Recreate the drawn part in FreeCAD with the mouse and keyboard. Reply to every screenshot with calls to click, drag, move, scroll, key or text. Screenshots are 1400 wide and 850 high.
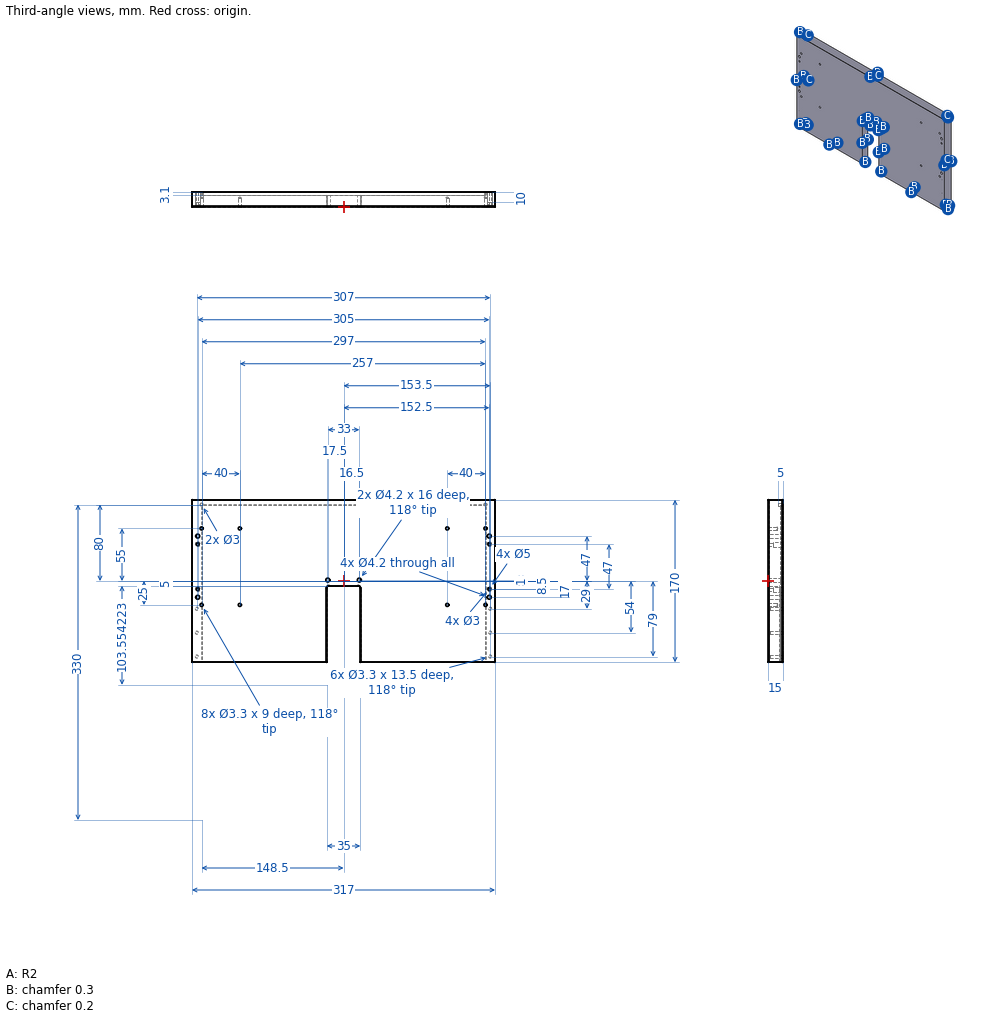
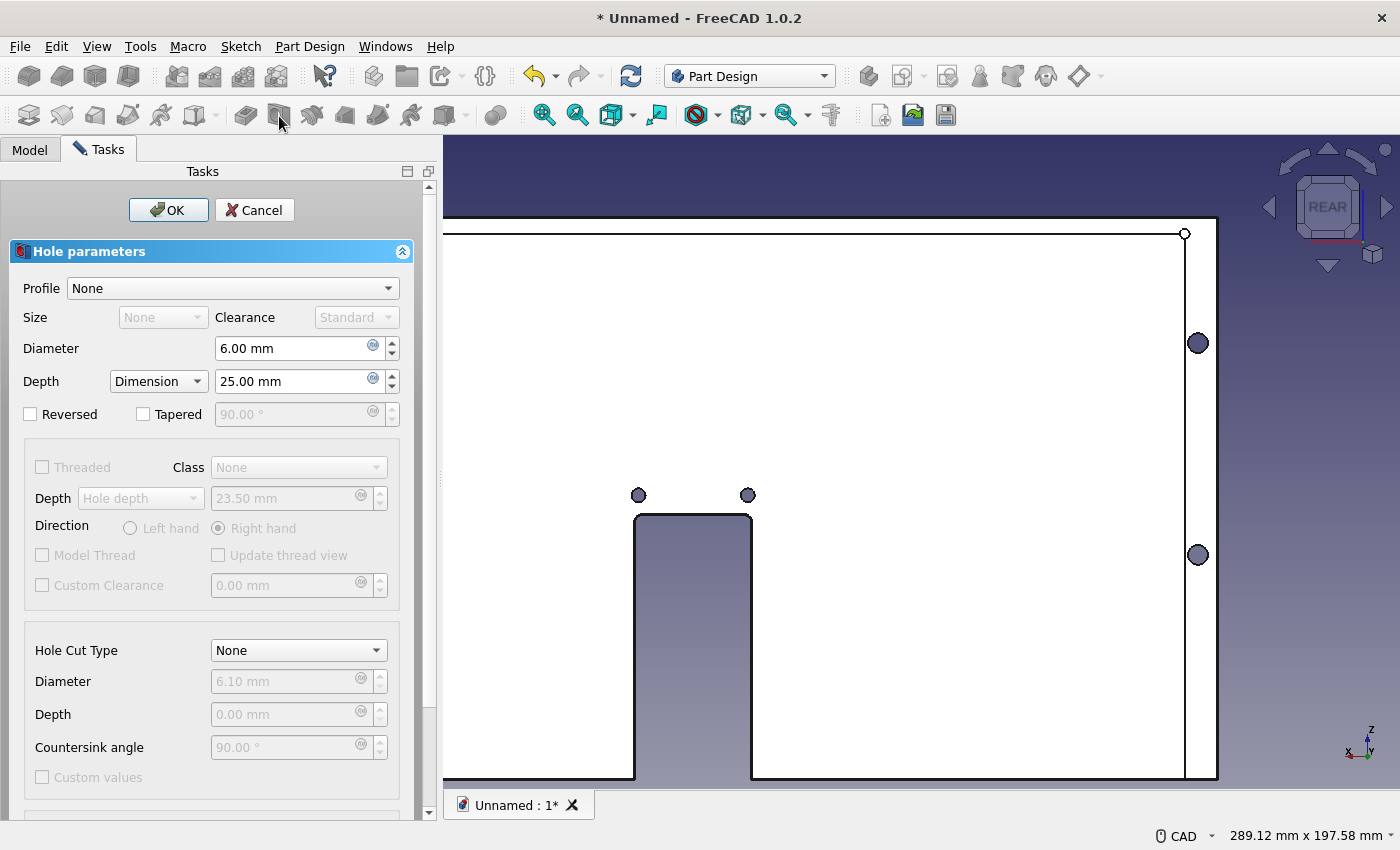
triple_click(300, 348)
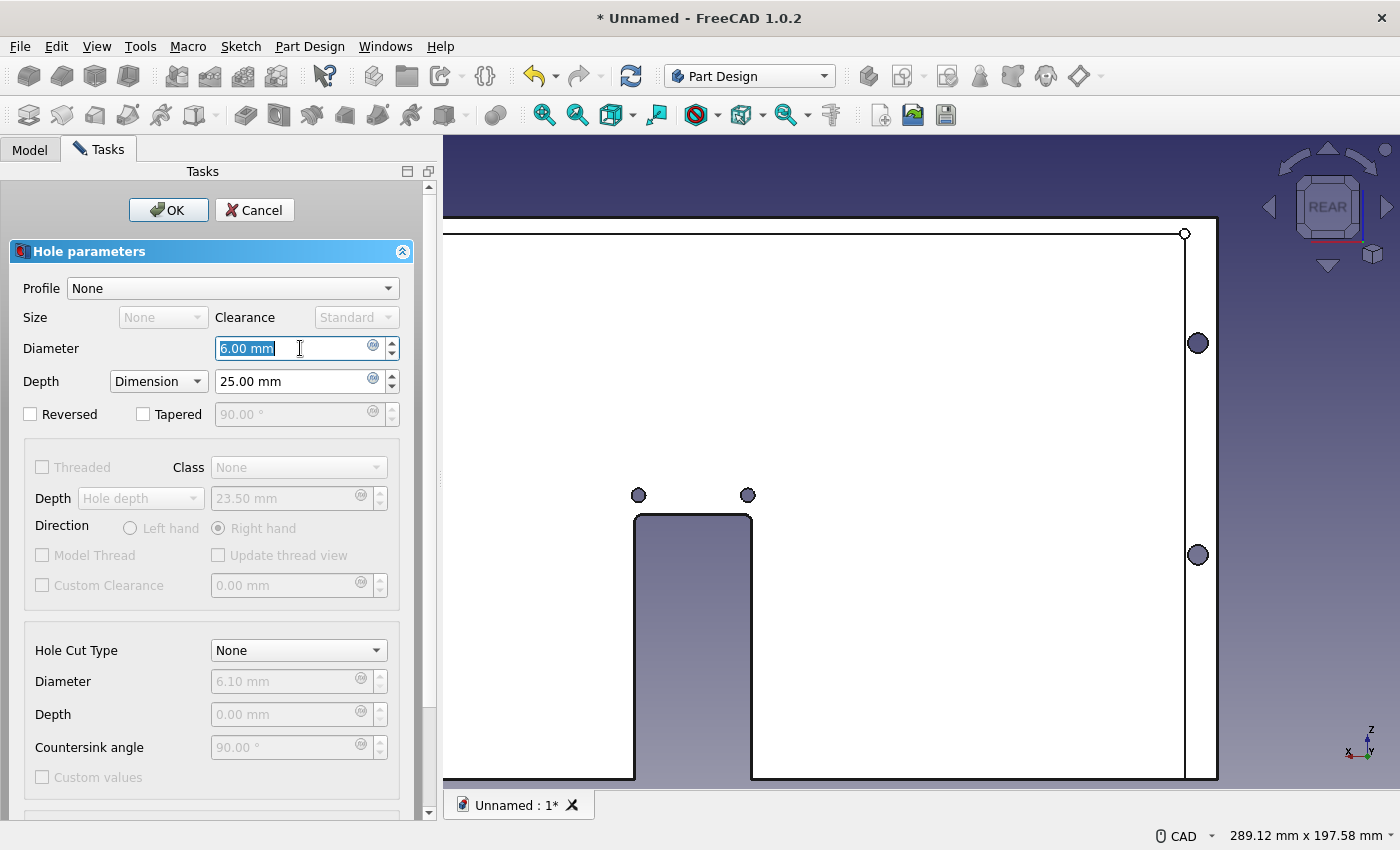
text(4.2)
key(Tab)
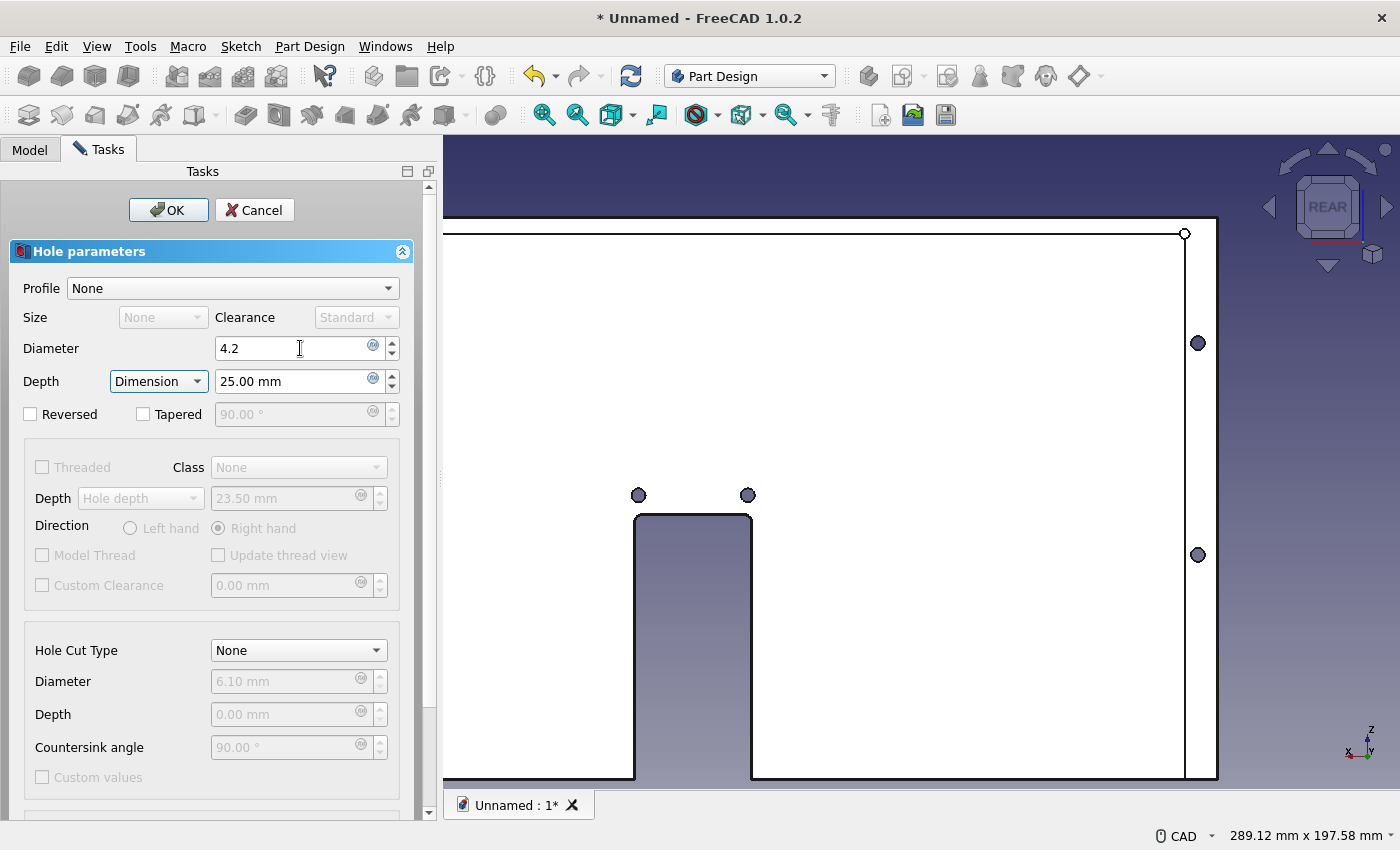
click(160, 382)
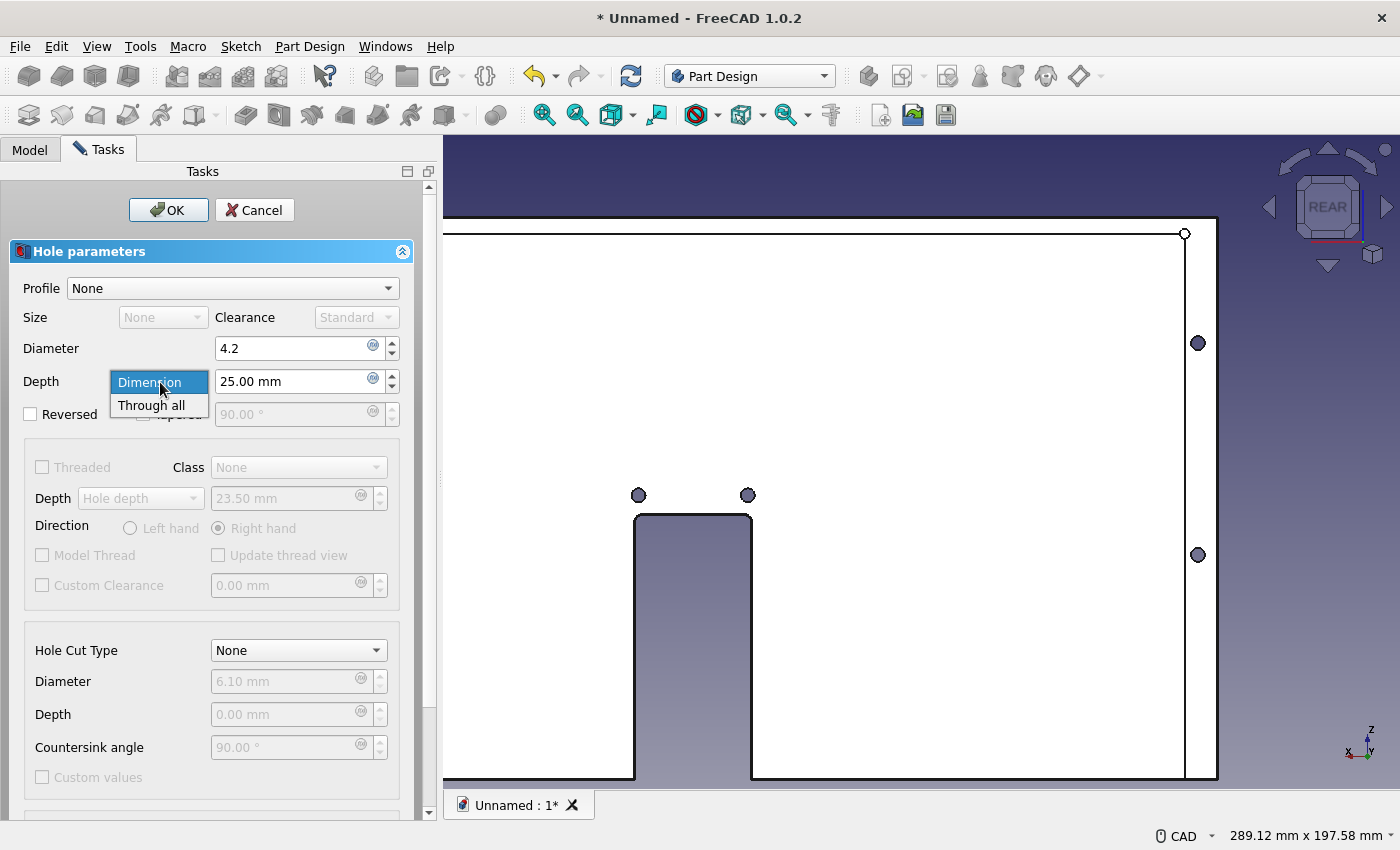
click(158, 406)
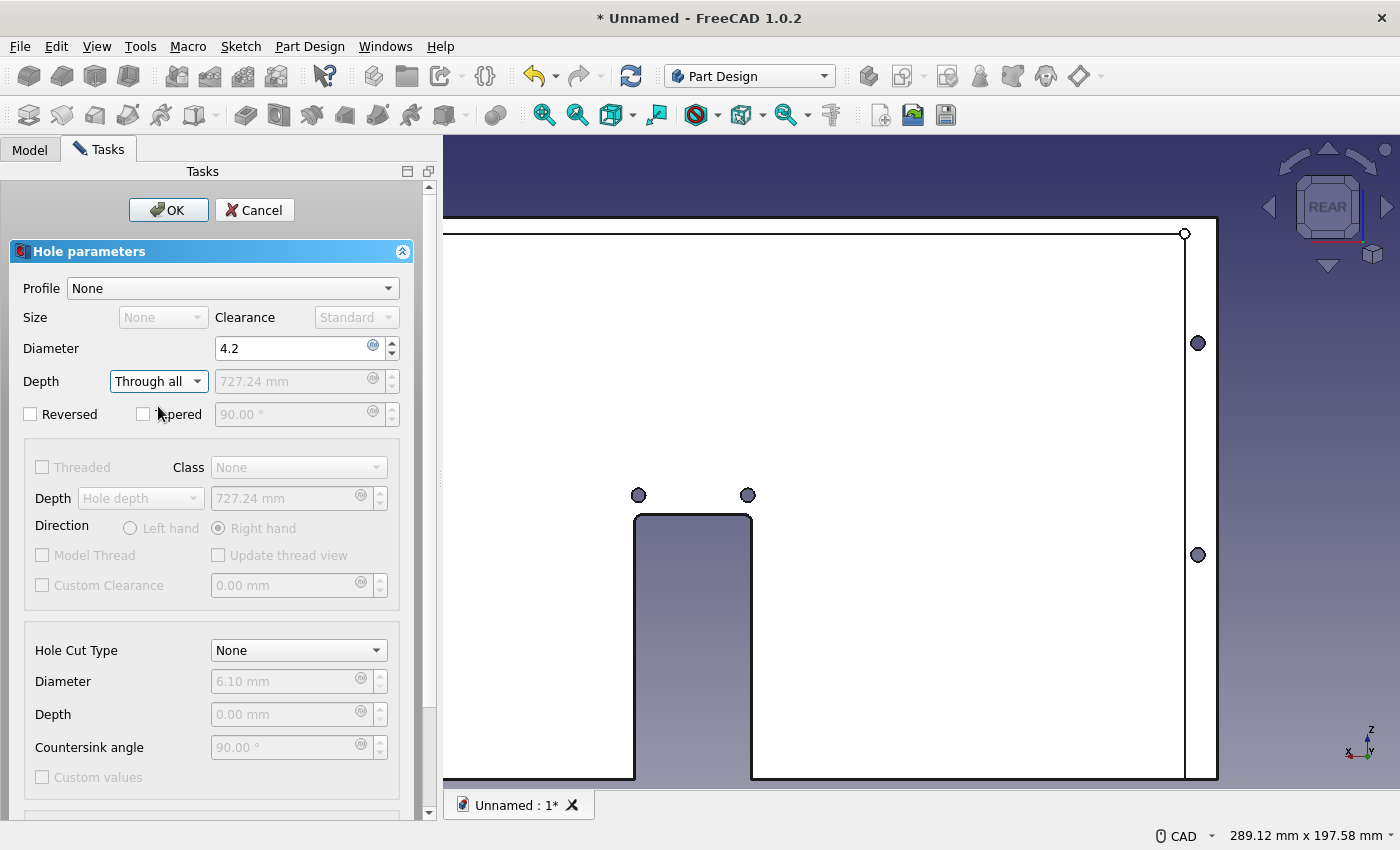
click(169, 210)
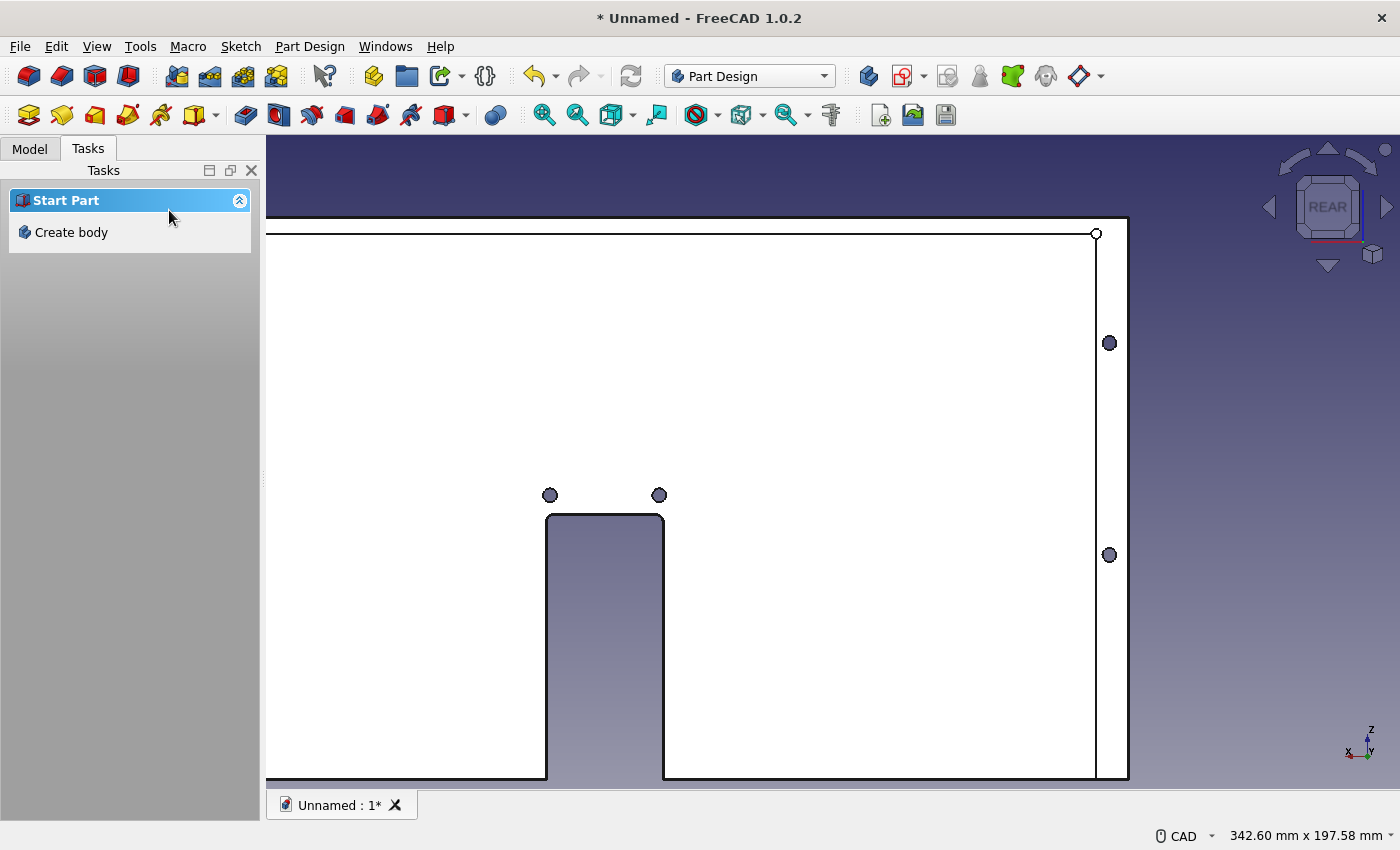
key(v)
key(f)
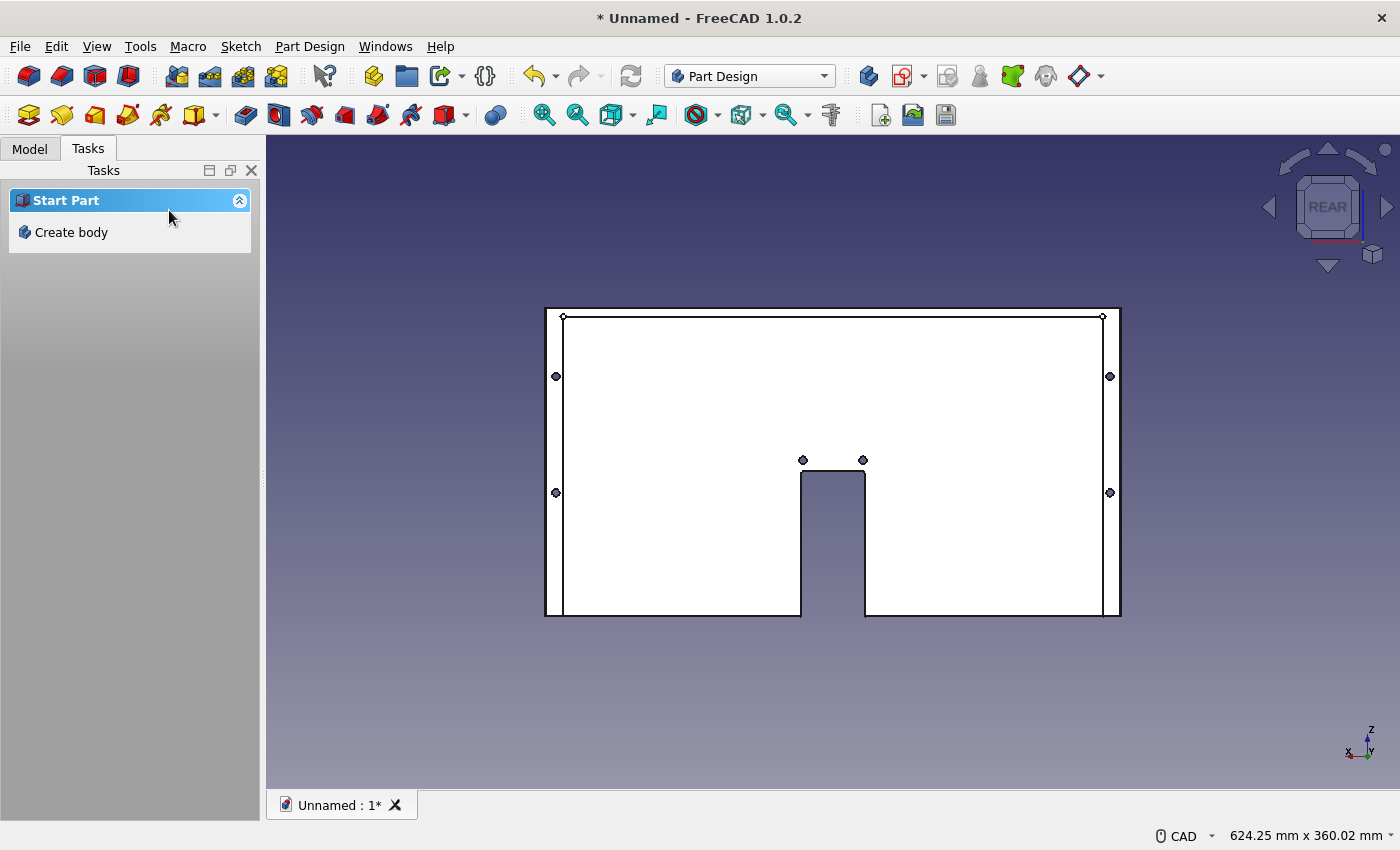
click(1111, 452)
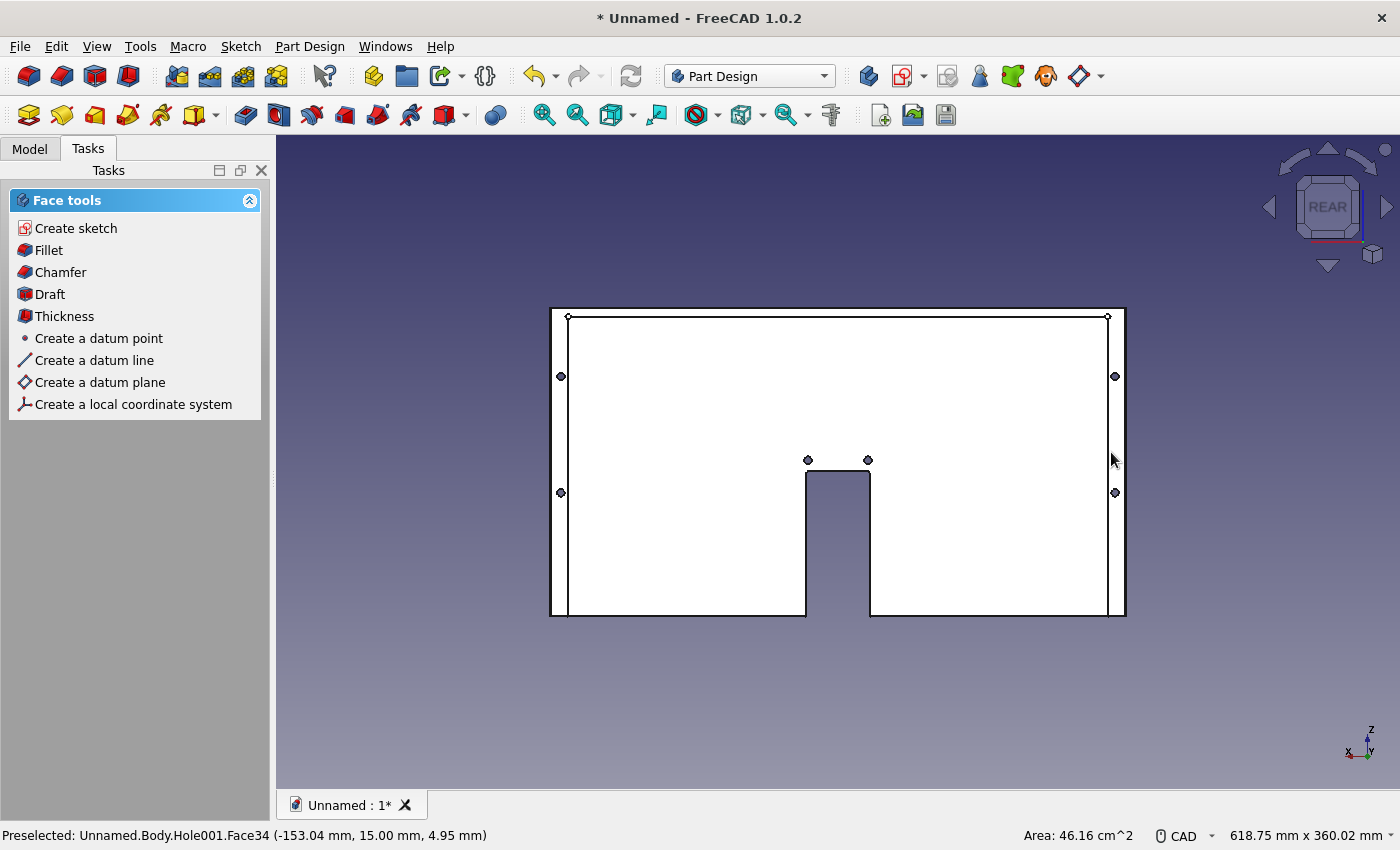
click(902, 76)